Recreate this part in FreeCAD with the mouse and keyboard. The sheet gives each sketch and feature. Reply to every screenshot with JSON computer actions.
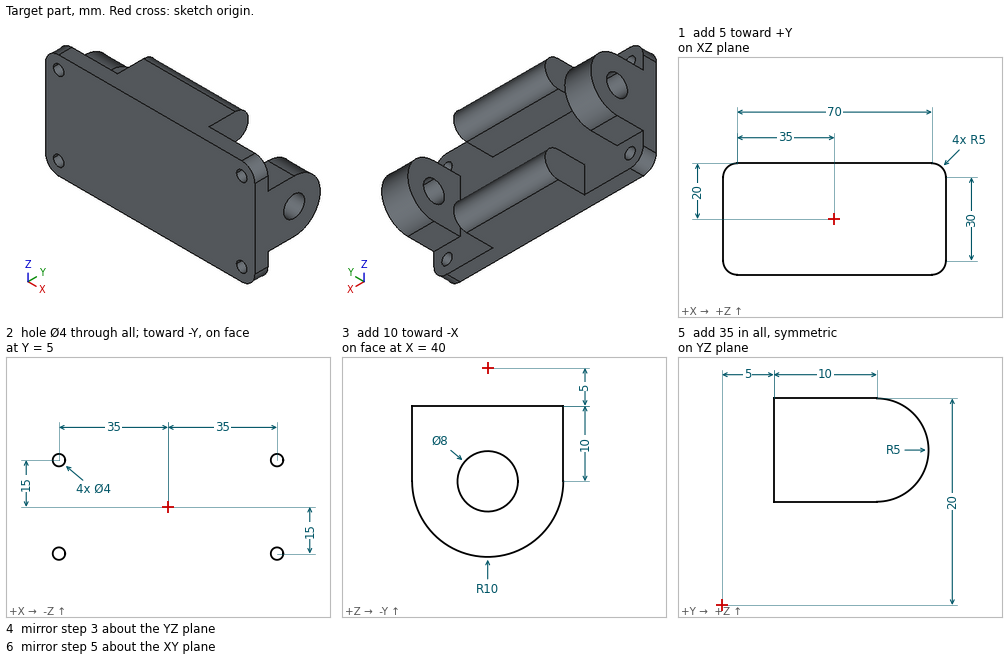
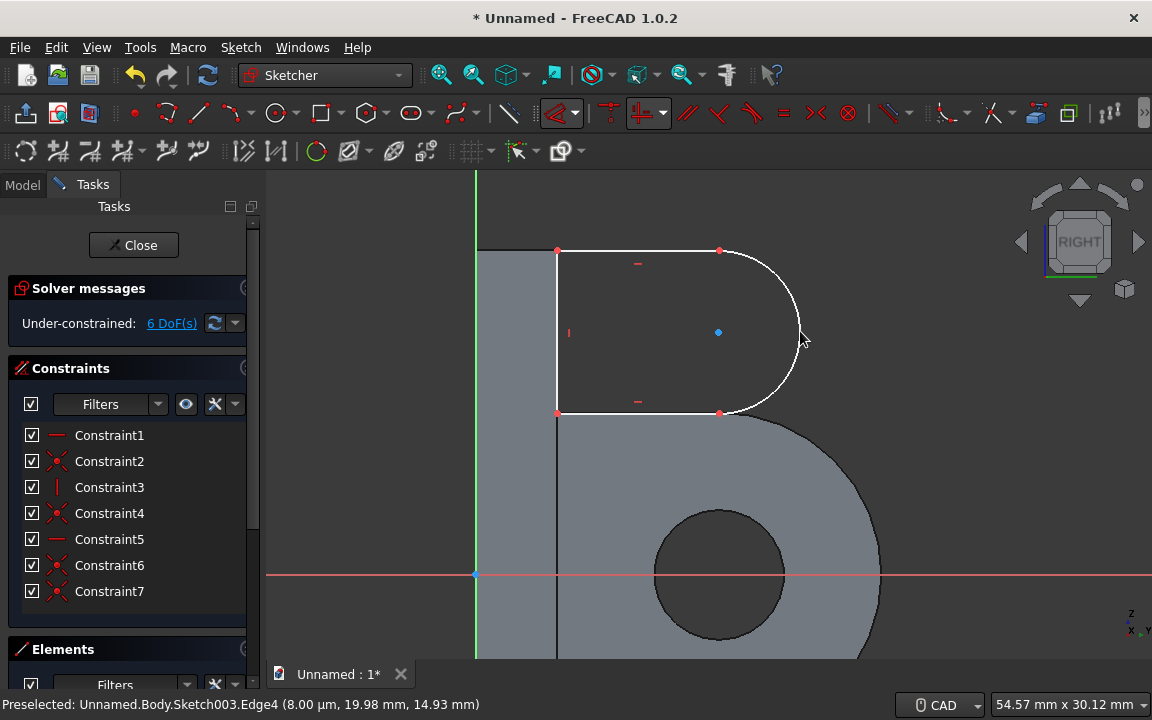
{"action": "left_click", "coordinate": [670, 251]}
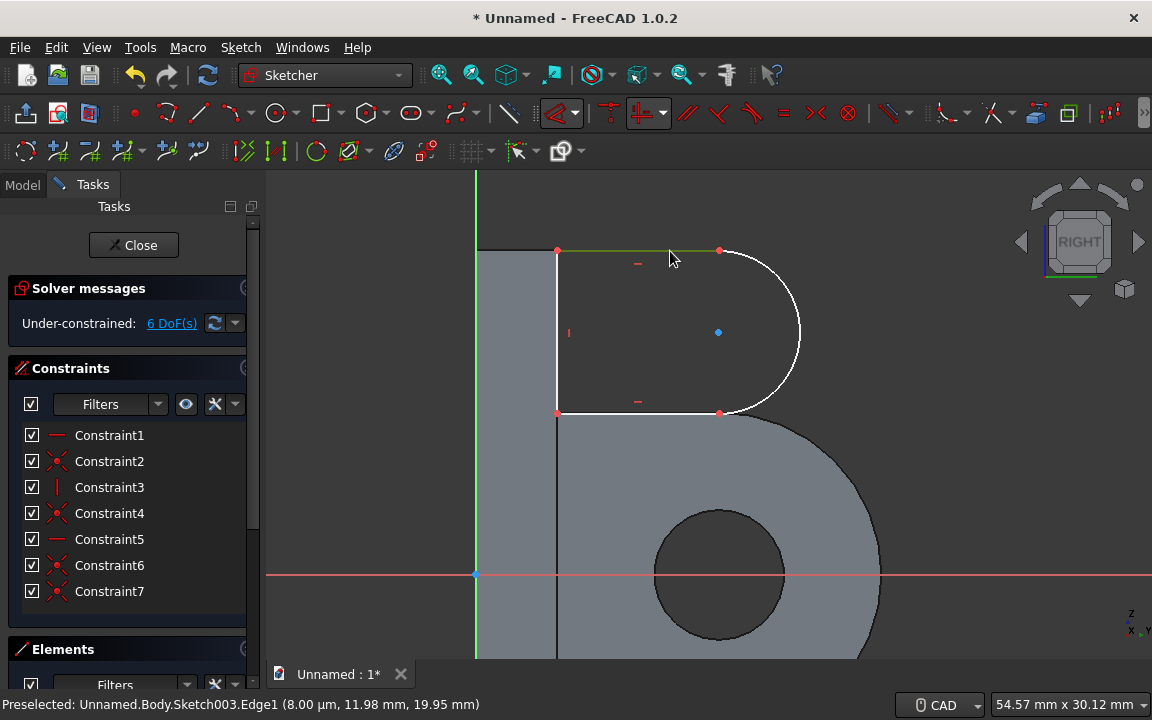
{"action": "left_click", "coordinate": [785, 380]}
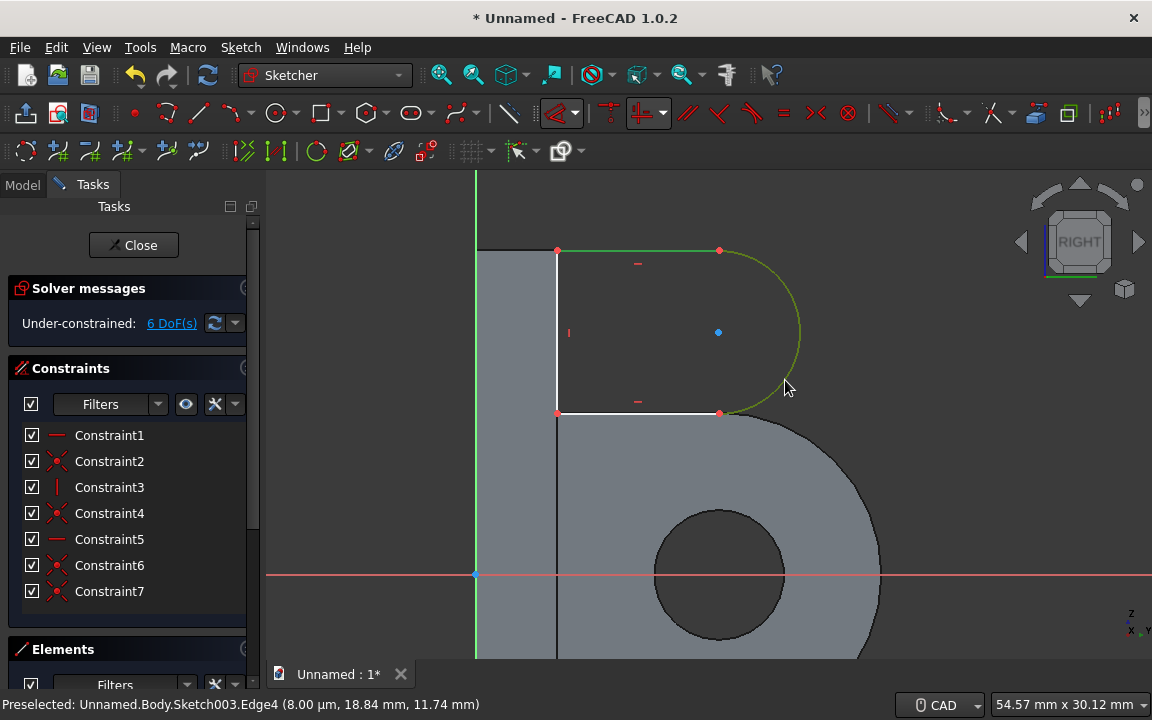
{"action": "left_click", "coordinate": [752, 114]}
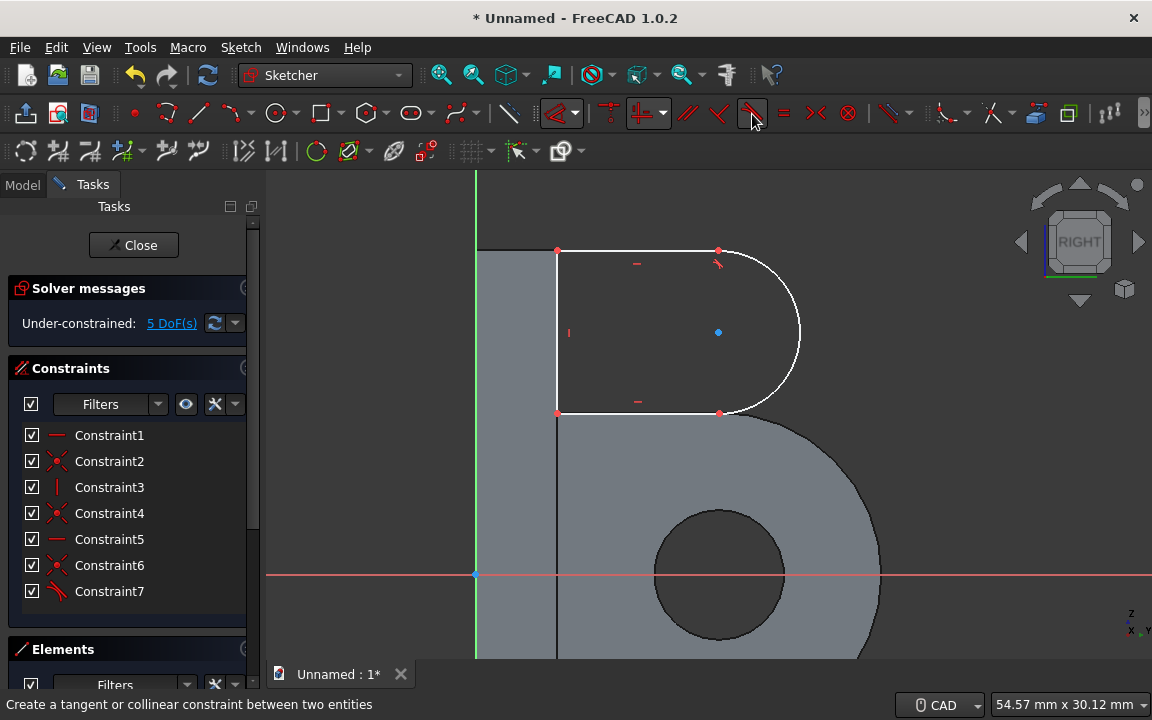
{"action": "left_click", "coordinate": [606, 414]}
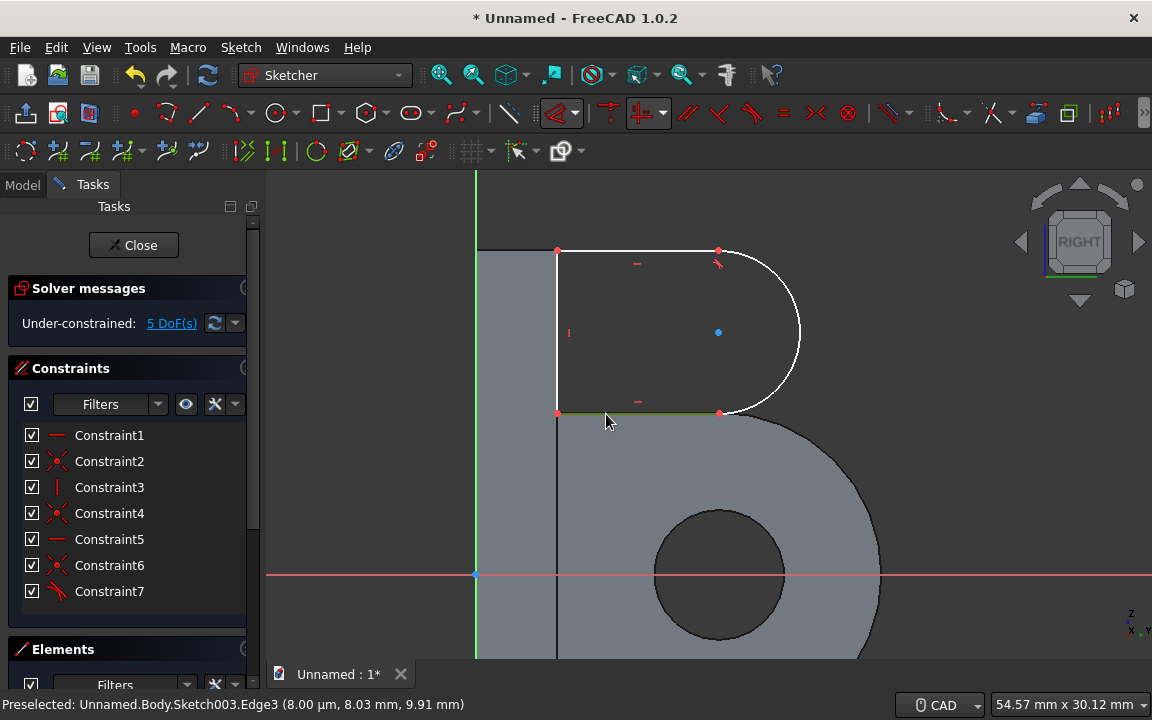
{"action": "left_click", "coordinate": [785, 380]}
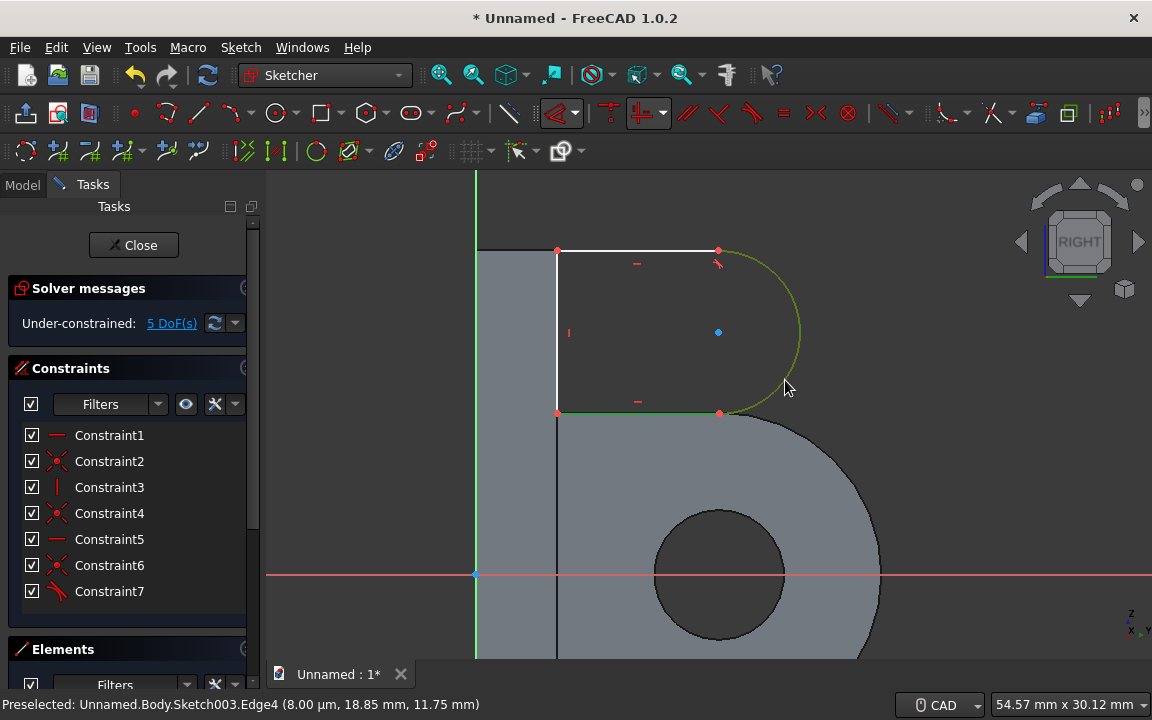
{"action": "key", "text": "t"}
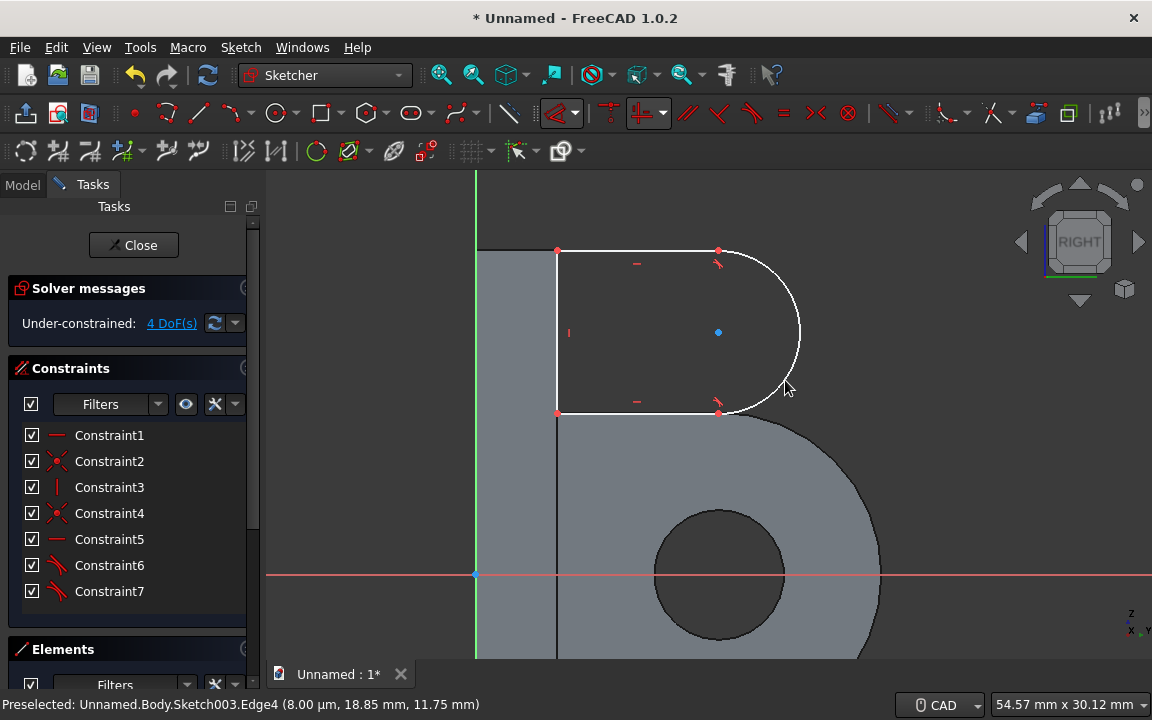
{"action": "left_click", "coordinate": [784, 380]}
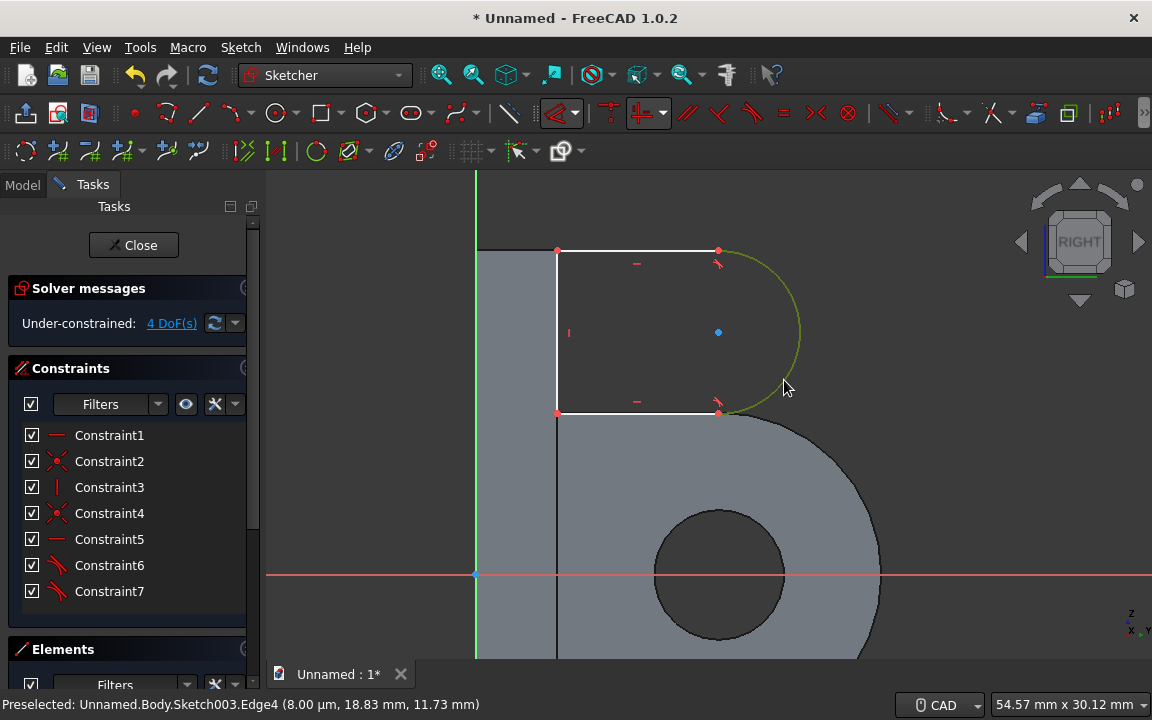
{"action": "key", "text": "k r"}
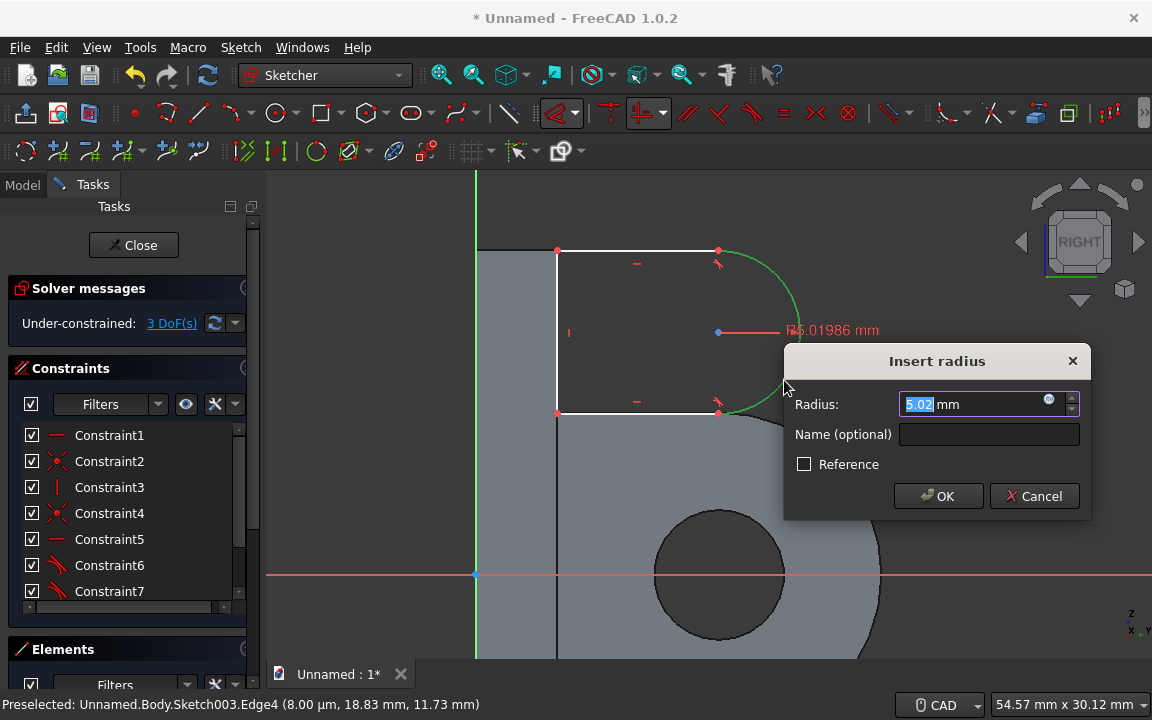
{"action": "type", "text": "5"}
{"action": "key", "text": "Return"}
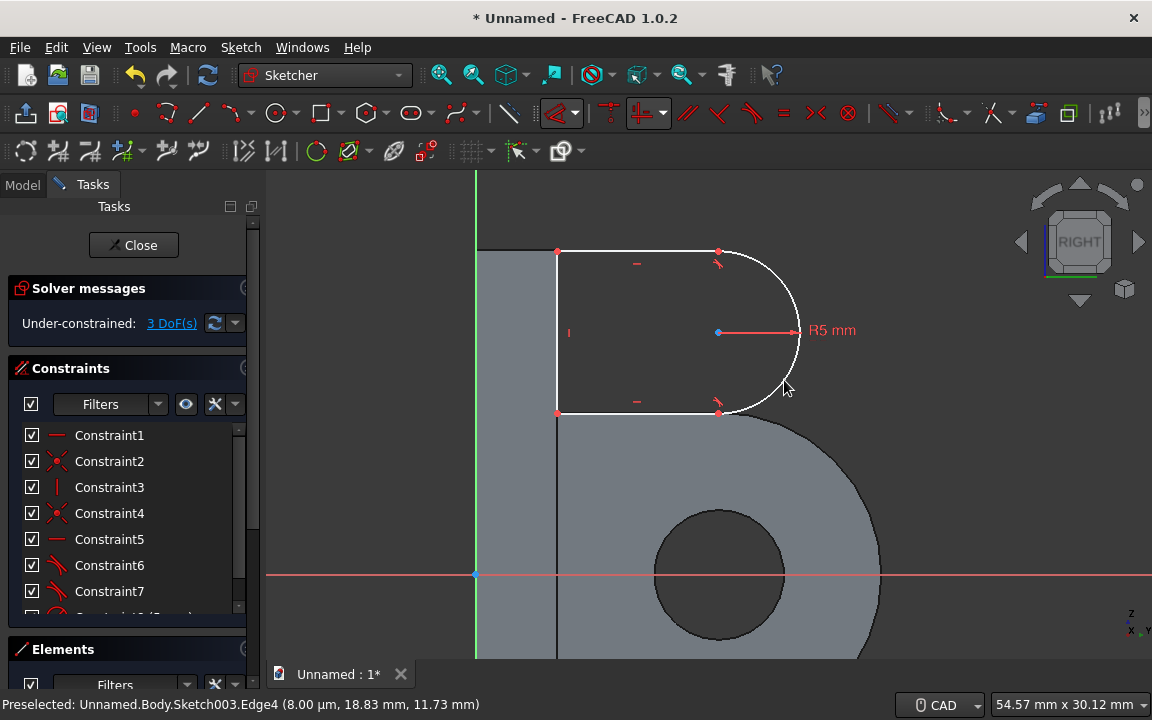
{"action": "left_click", "coordinate": [670, 251]}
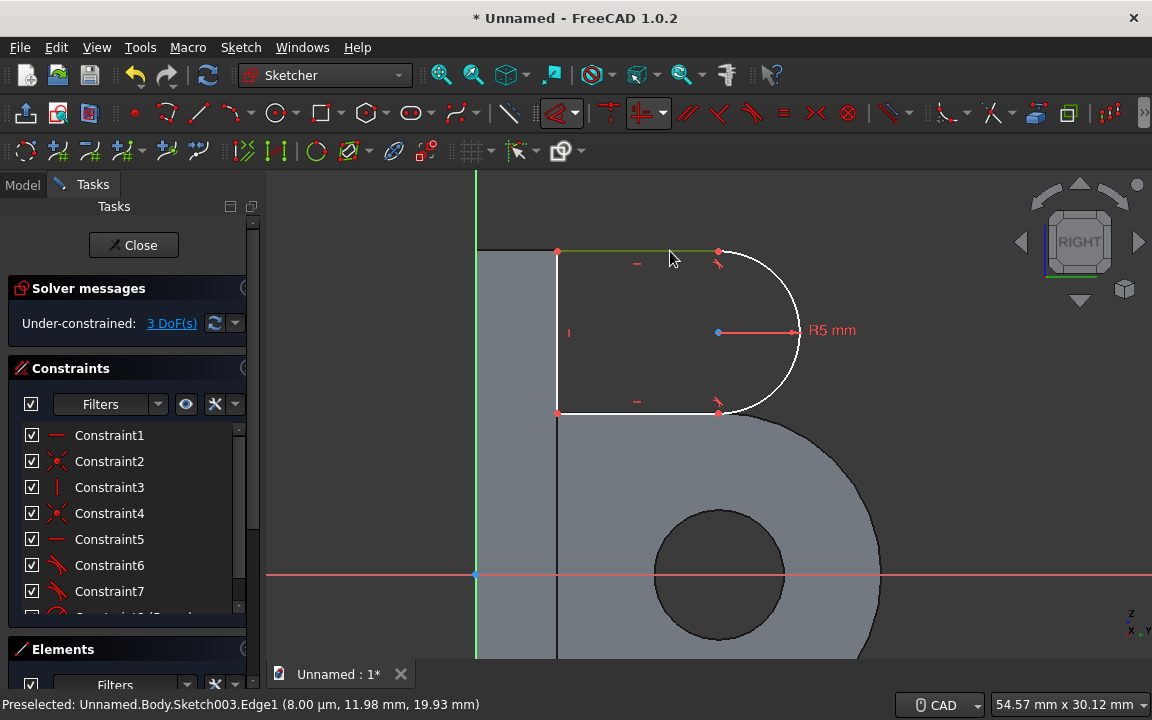
{"action": "left_click", "coordinate": [578, 114]}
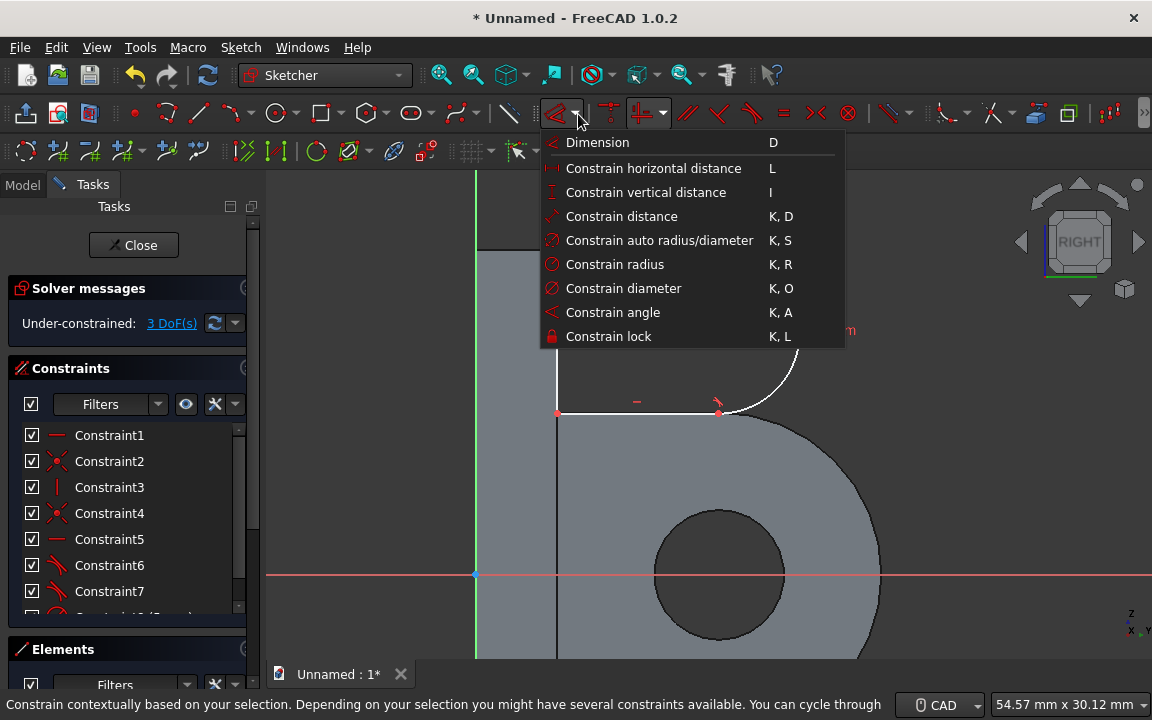
{"action": "left_click", "coordinate": [693, 168]}